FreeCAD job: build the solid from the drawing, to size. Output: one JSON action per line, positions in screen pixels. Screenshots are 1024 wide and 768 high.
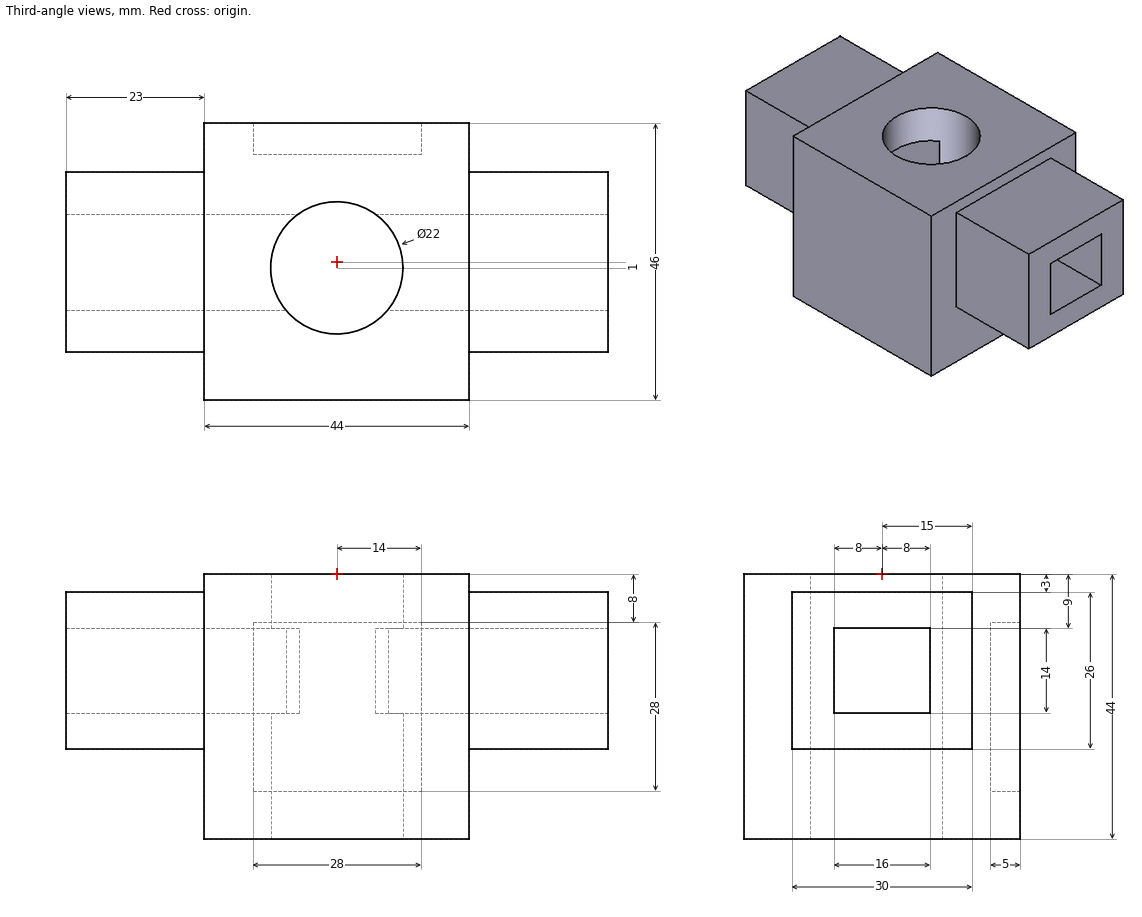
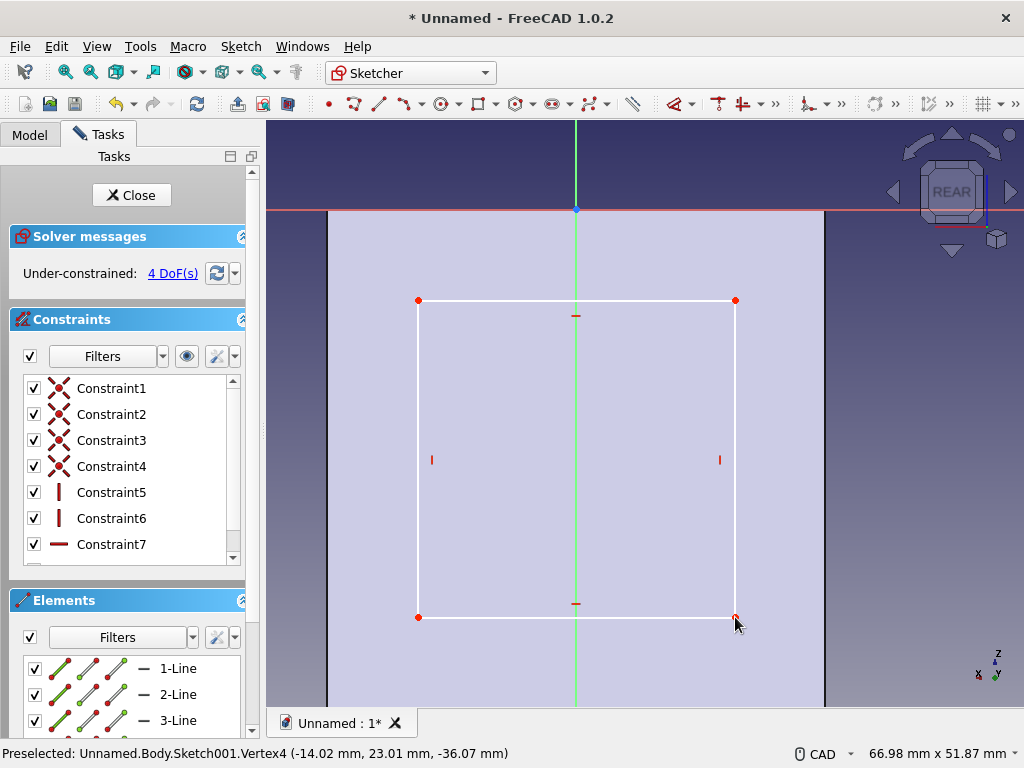
{"action": "left_click", "coordinate": [418, 396]}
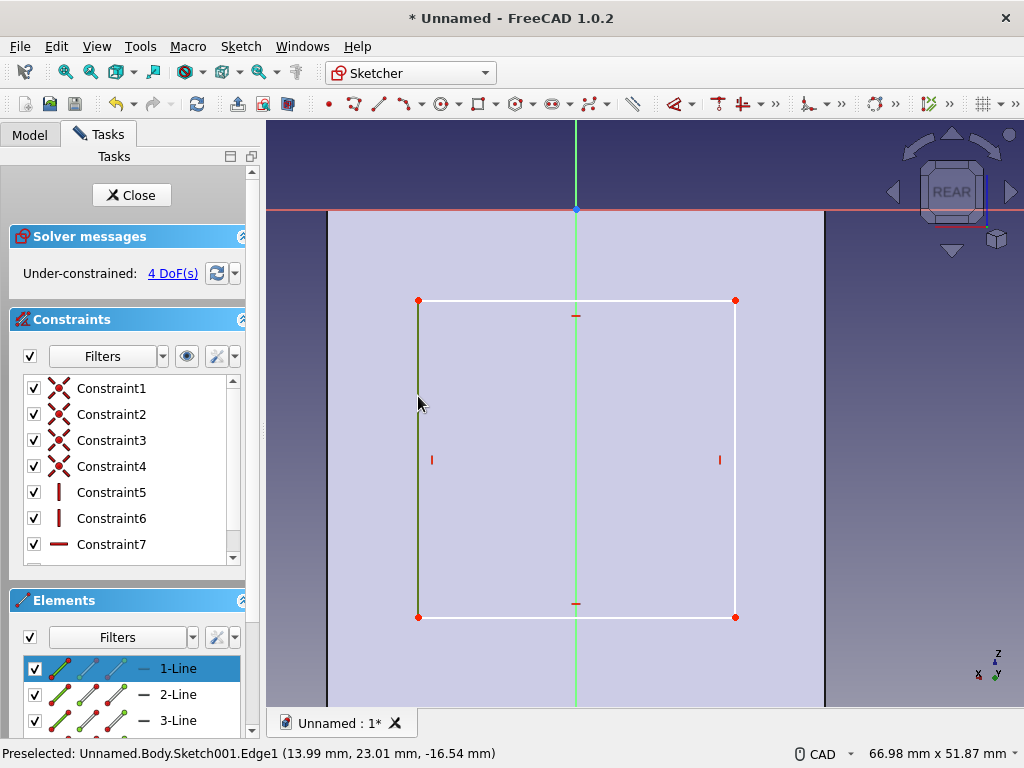
{"action": "left_click", "coordinate": [692, 104]}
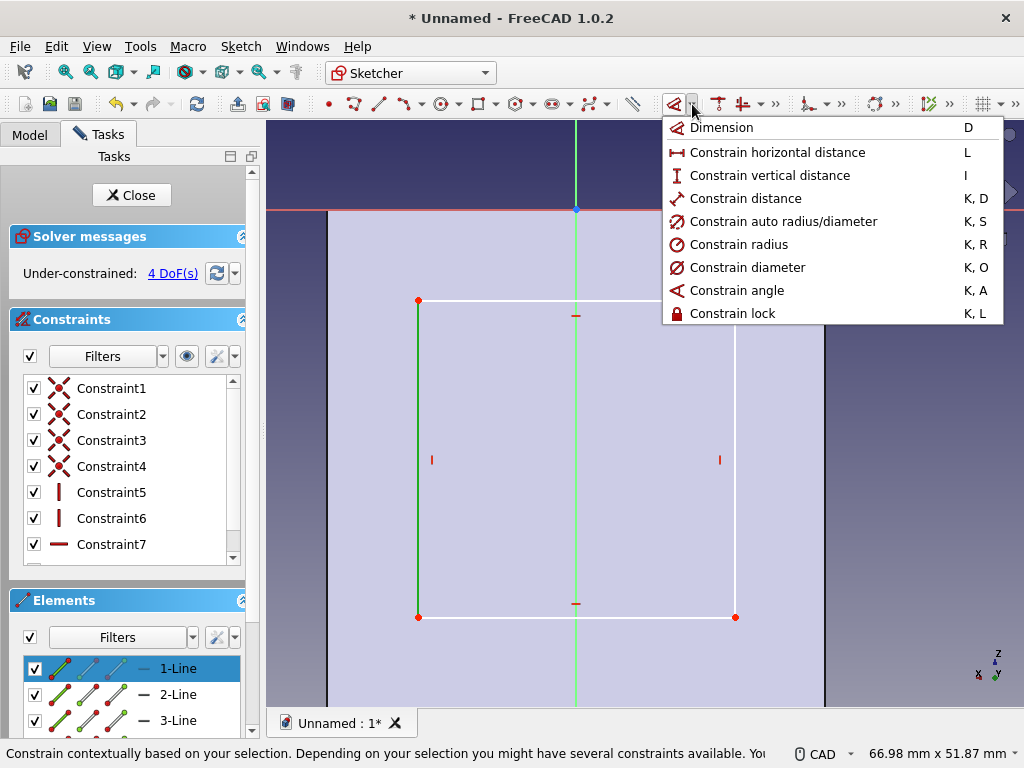
{"action": "left_click", "coordinate": [833, 176]}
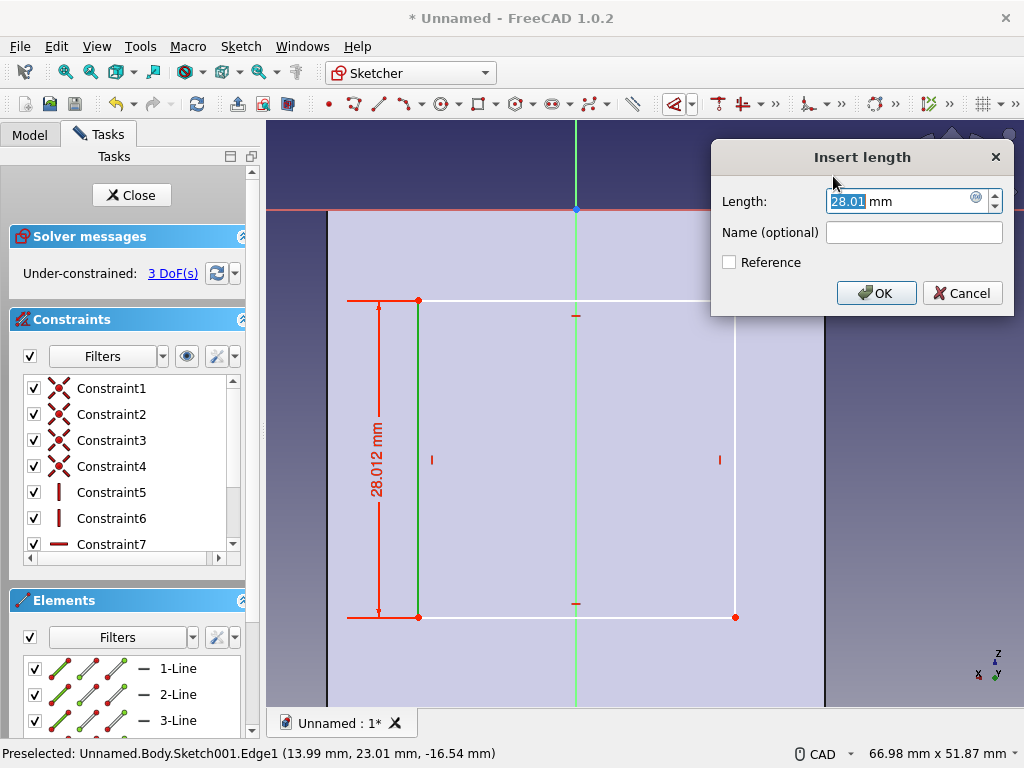
{"action": "type", "text": "28"}
{"action": "key", "text": "Return"}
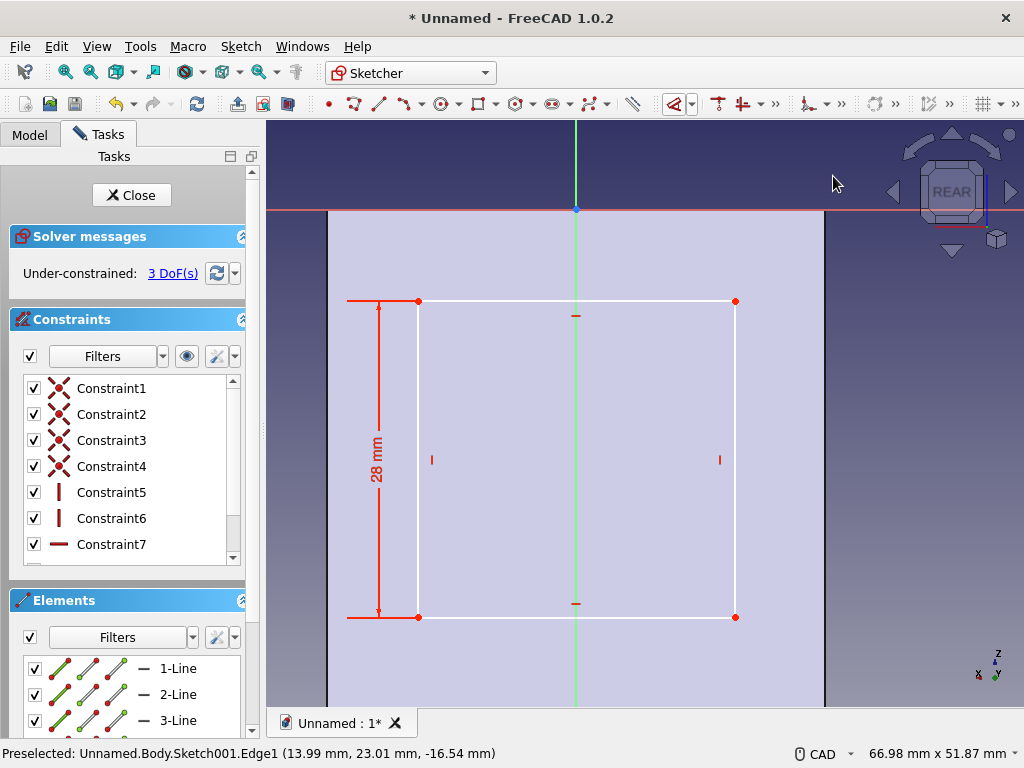
{"action": "left_click", "coordinate": [513, 618]}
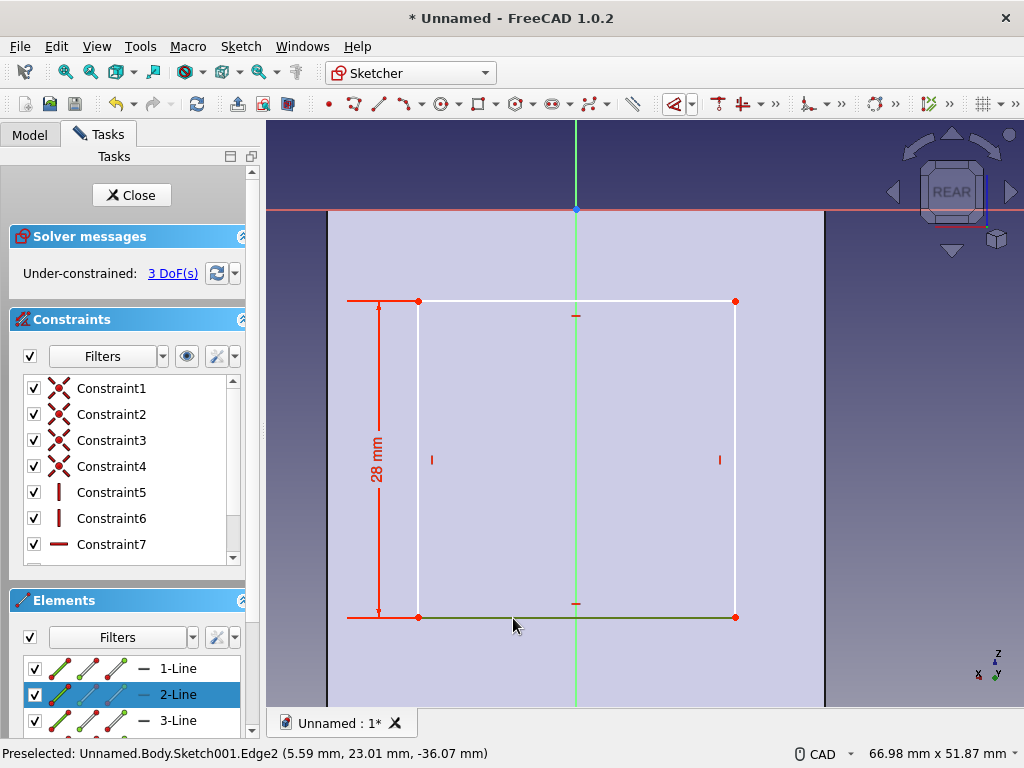
{"action": "key", "text": "l"}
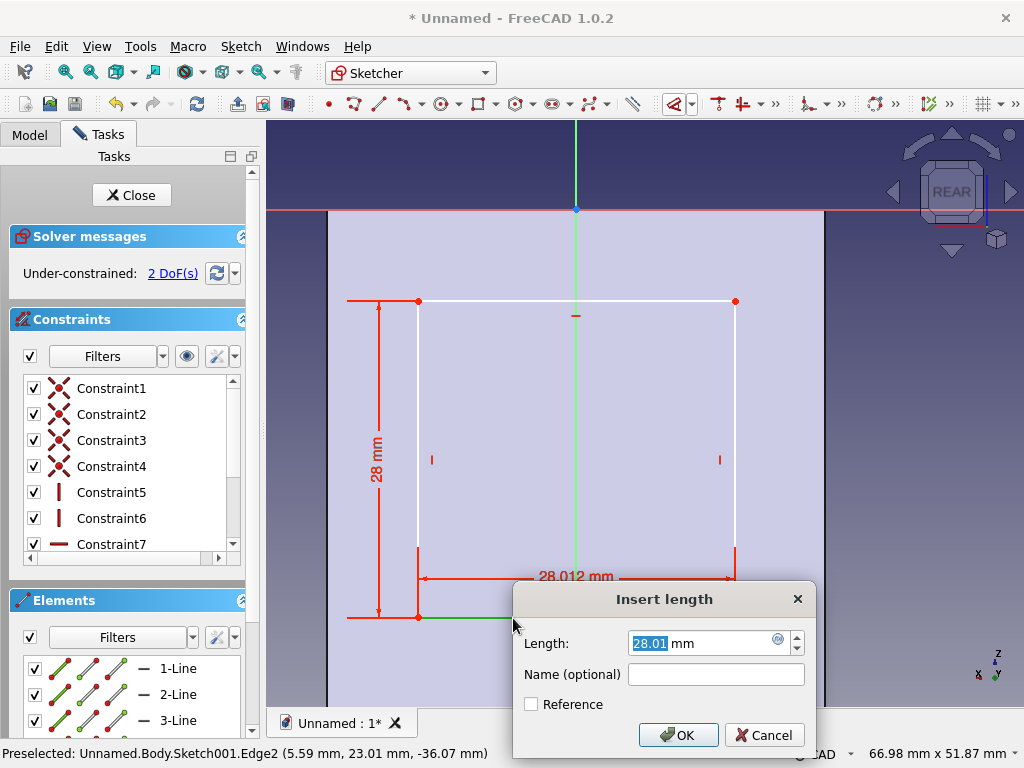
{"action": "type", "text": "28"}
{"action": "key", "text": "Return"}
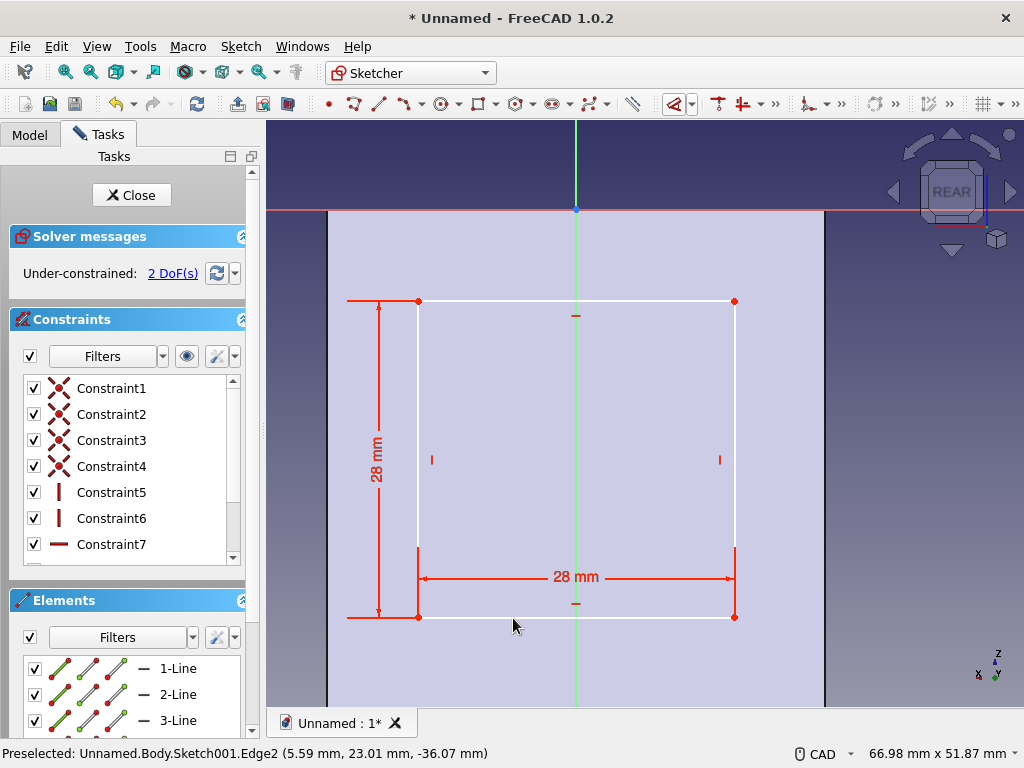
{"action": "left_click", "coordinate": [418, 301]}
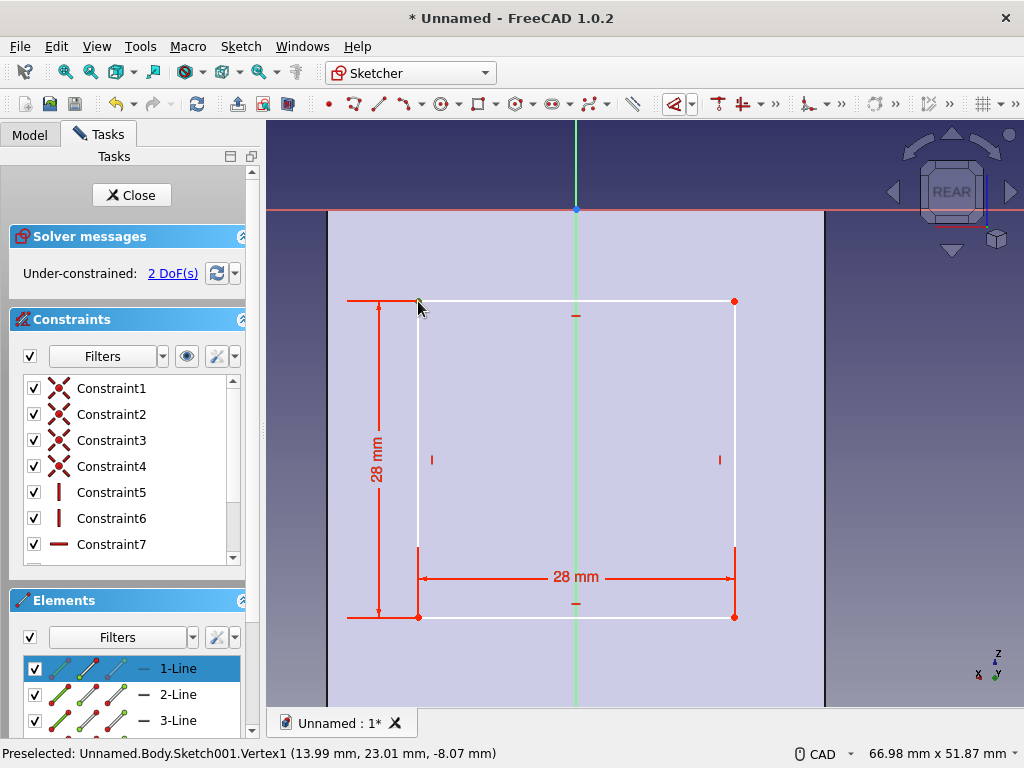
{"action": "key", "text": "i"}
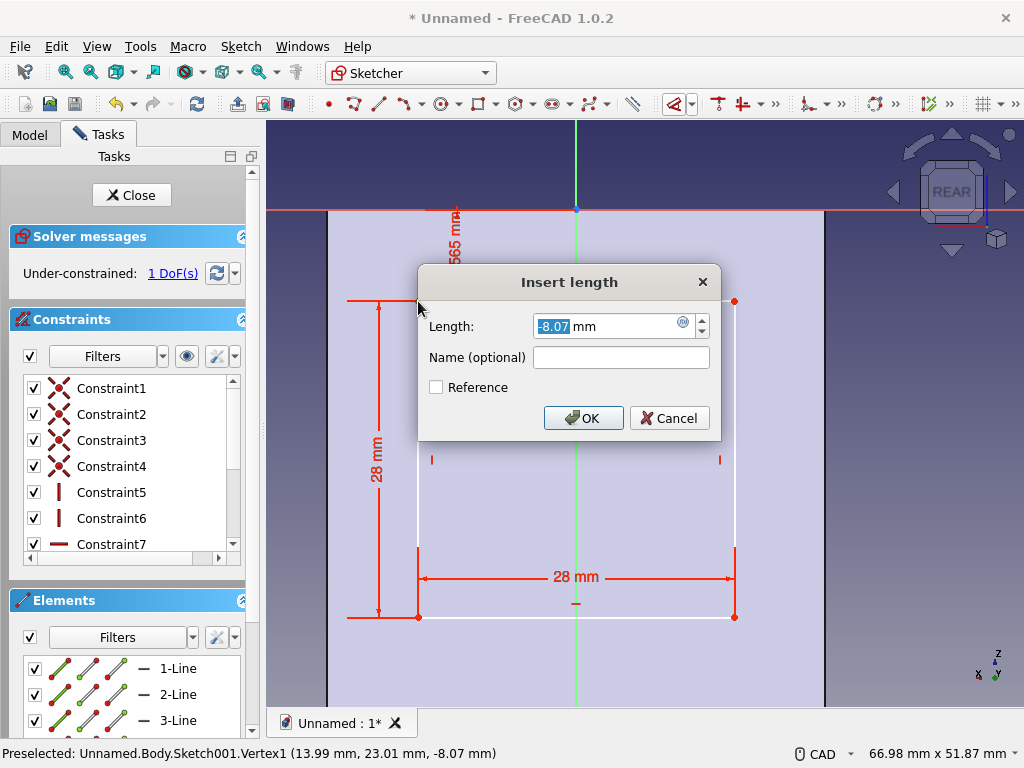
{"action": "type", "text": "-8"}
{"action": "key", "text": "Return"}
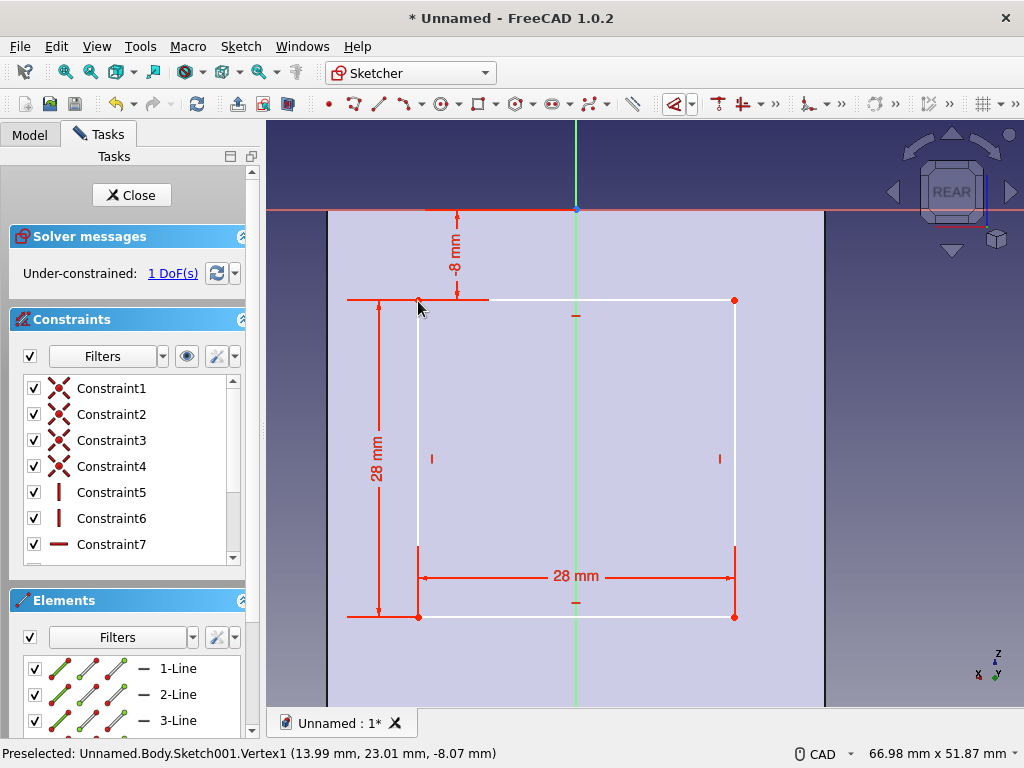
{"action": "left_click", "coordinate": [418, 300]}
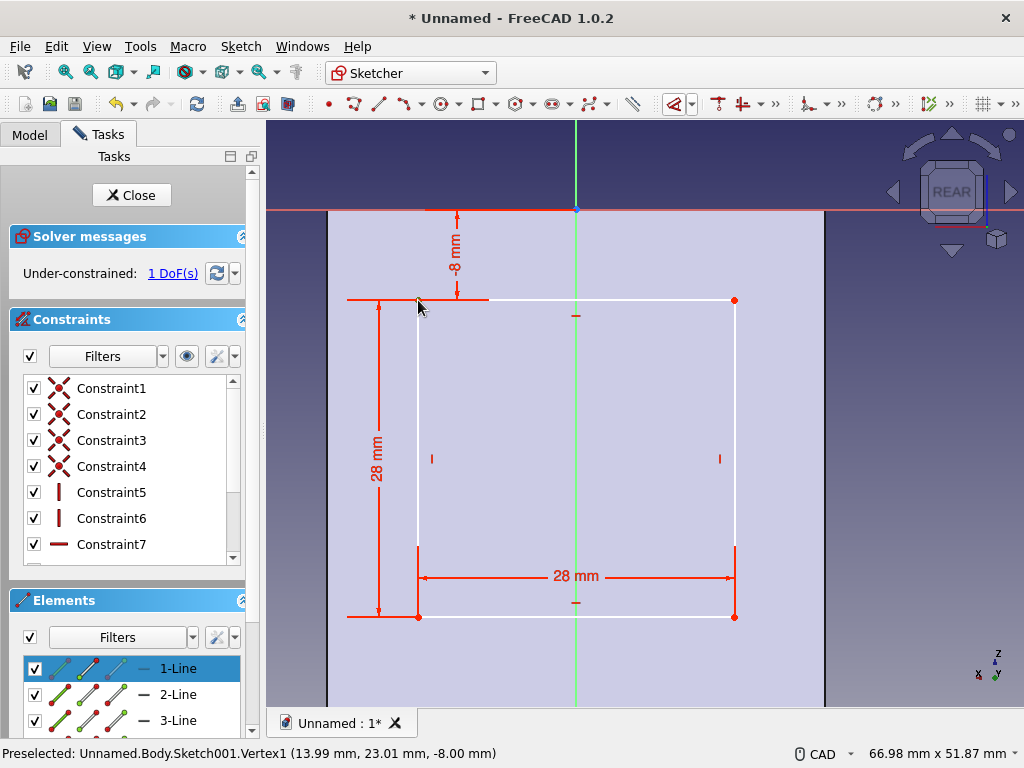
{"action": "key", "text": "l"}